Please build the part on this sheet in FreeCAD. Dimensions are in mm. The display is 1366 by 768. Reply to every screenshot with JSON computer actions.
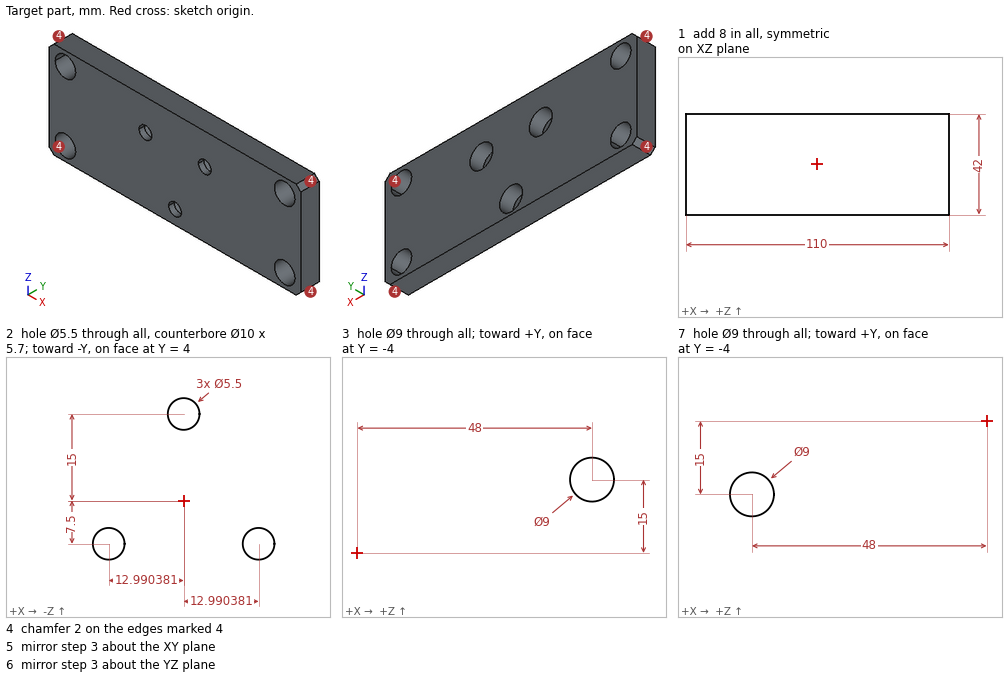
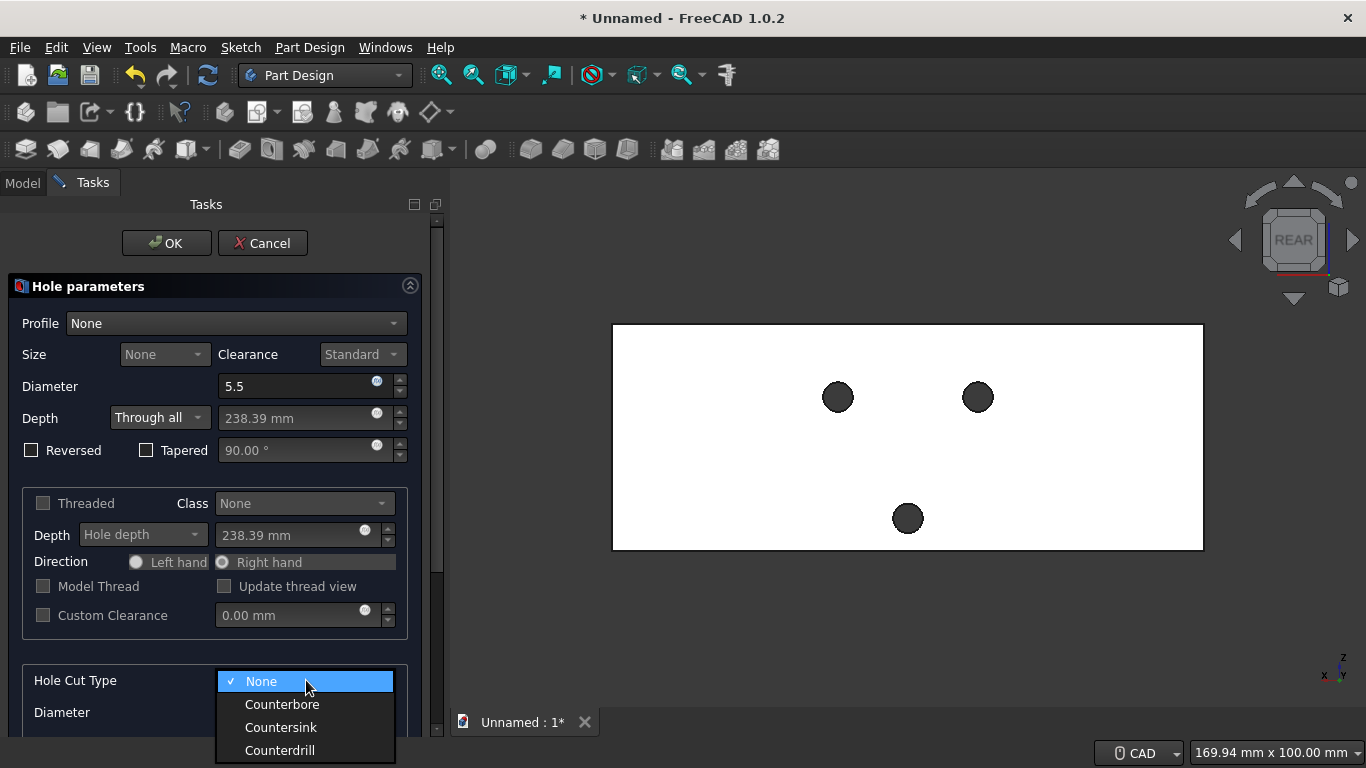
{"action": "left_click", "coordinate": [304, 704]}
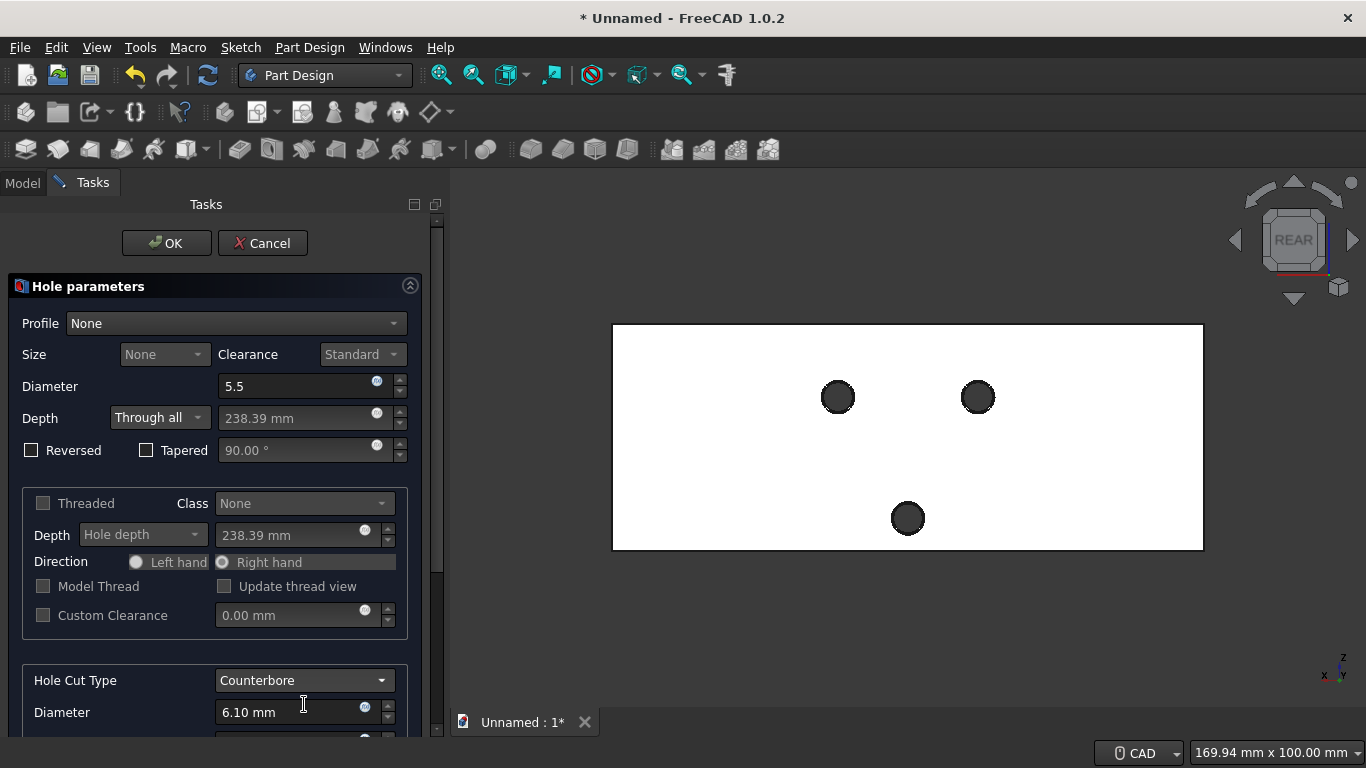
{"action": "triple_click", "coordinate": [298, 712]}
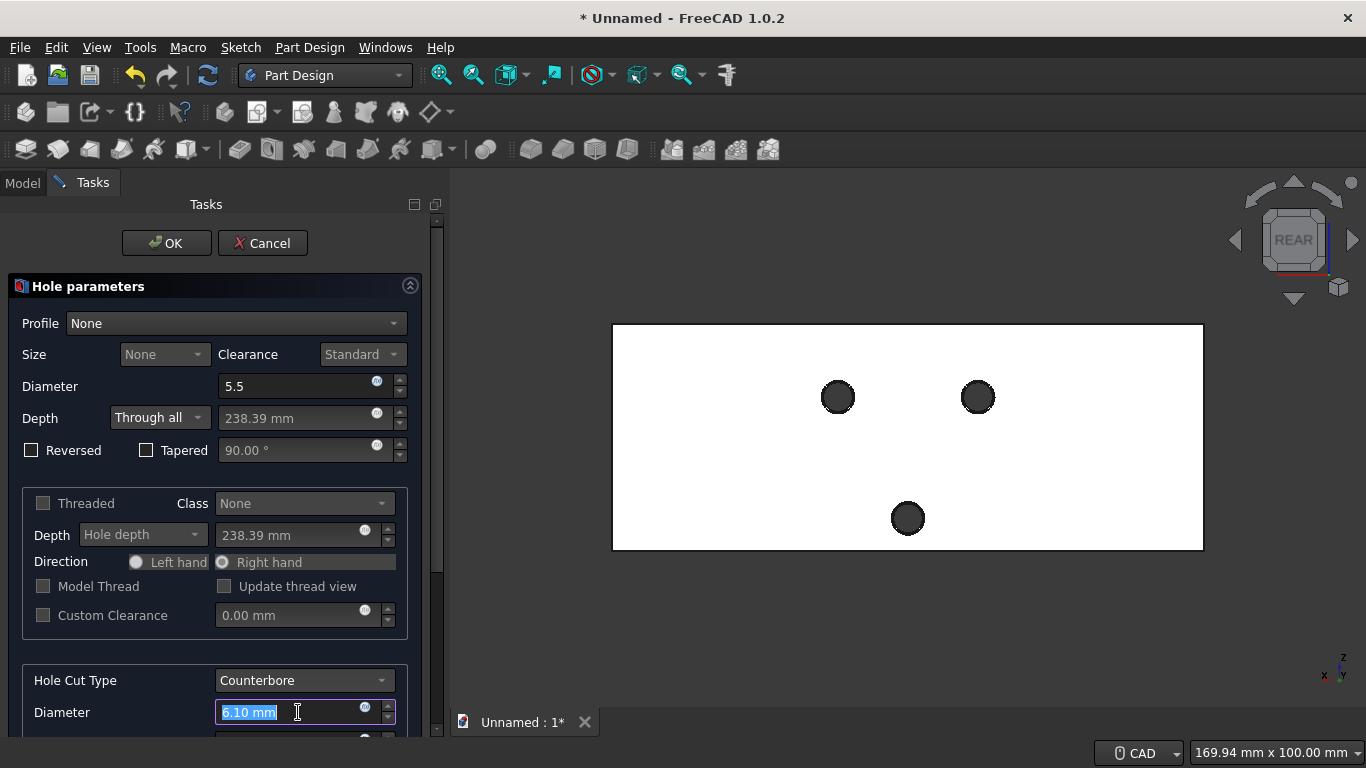
{"action": "type", "text": "10"}
{"action": "key", "text": "Tab"}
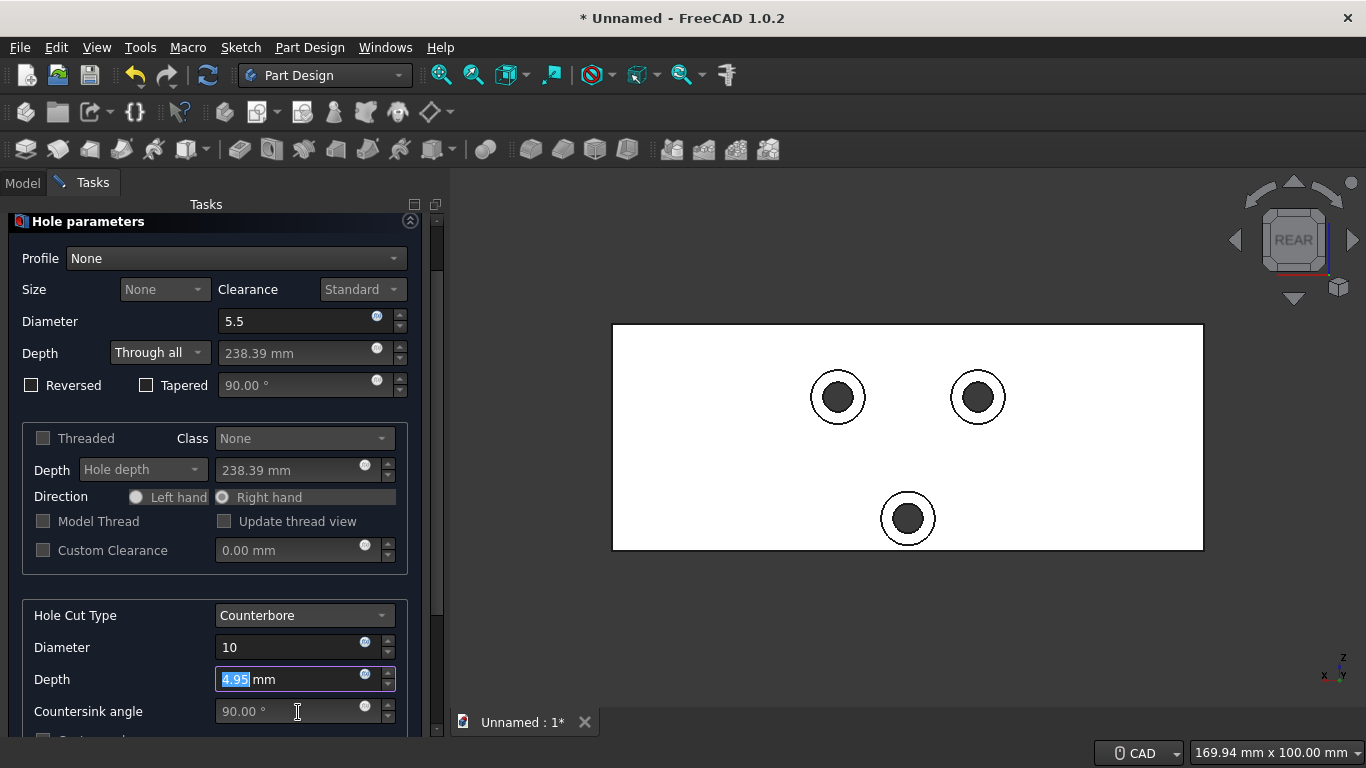
{"action": "type", "text": "5.7"}
{"action": "key", "text": "Tab"}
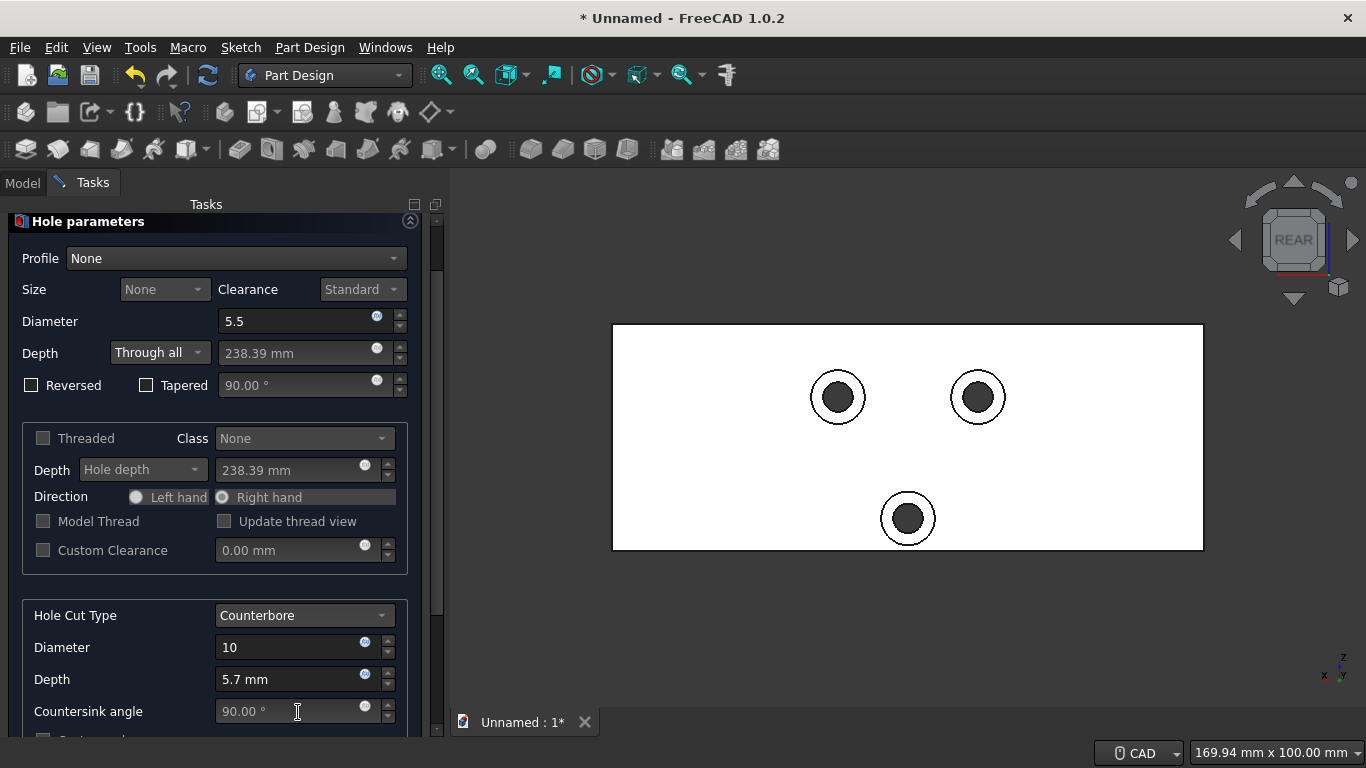
{"action": "scroll", "coordinate": [437, 475], "scroll_direction": "up", "scroll_amount": 2}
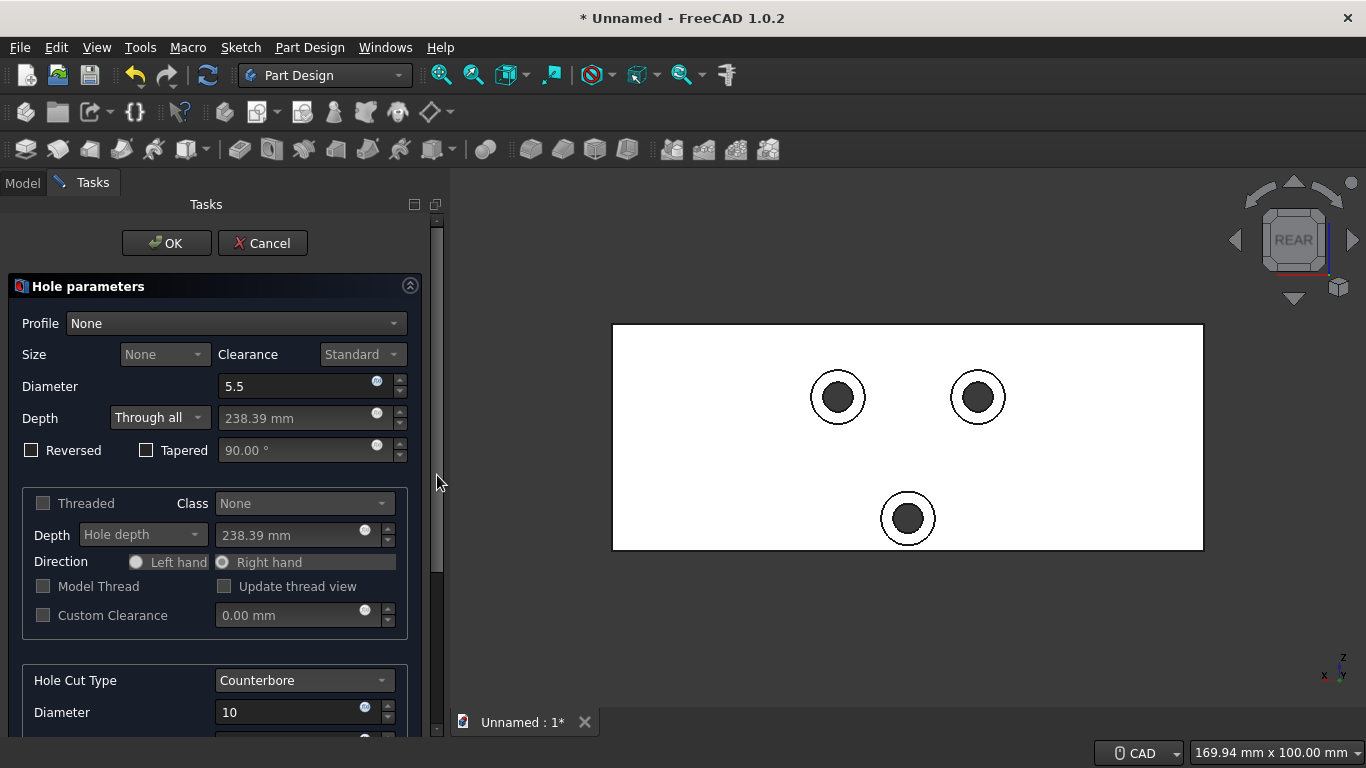
{"action": "left_click", "coordinate": [167, 243]}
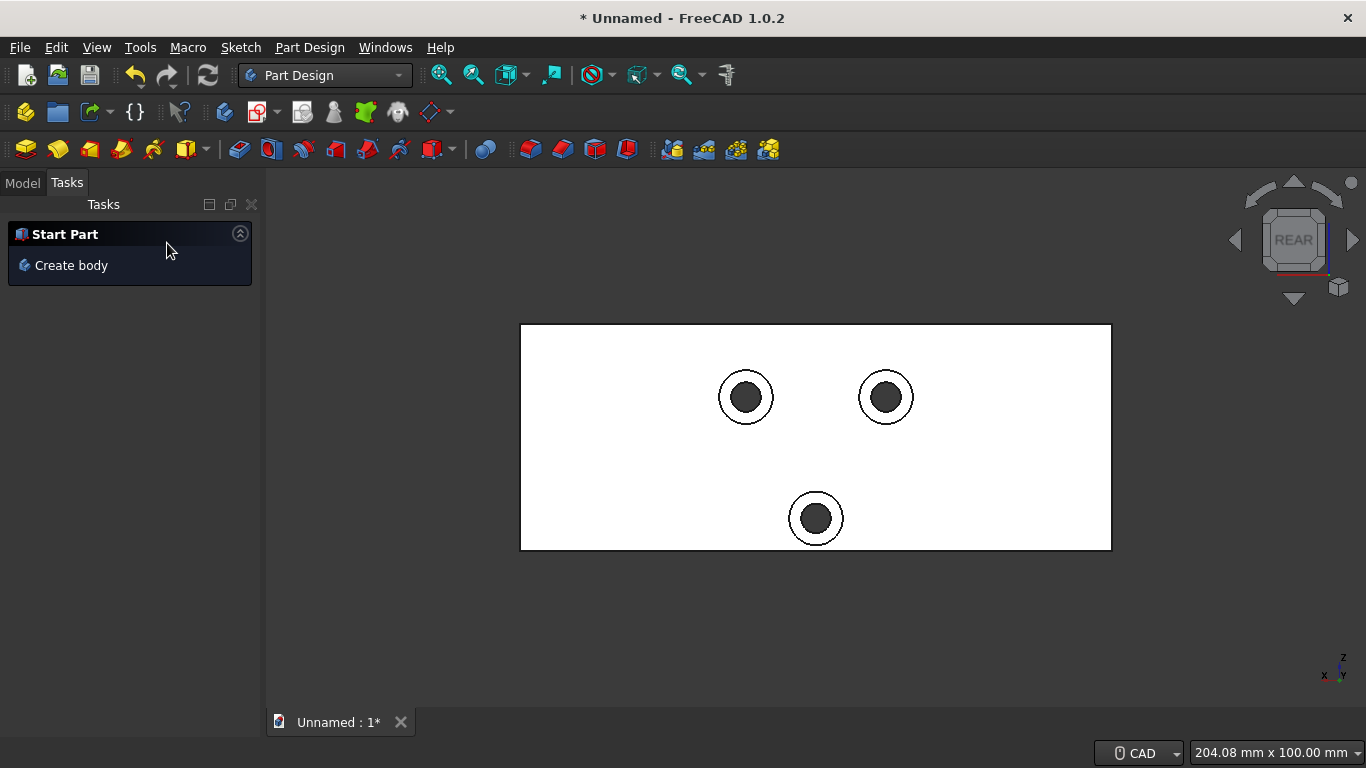
{"action": "key", "text": "0"}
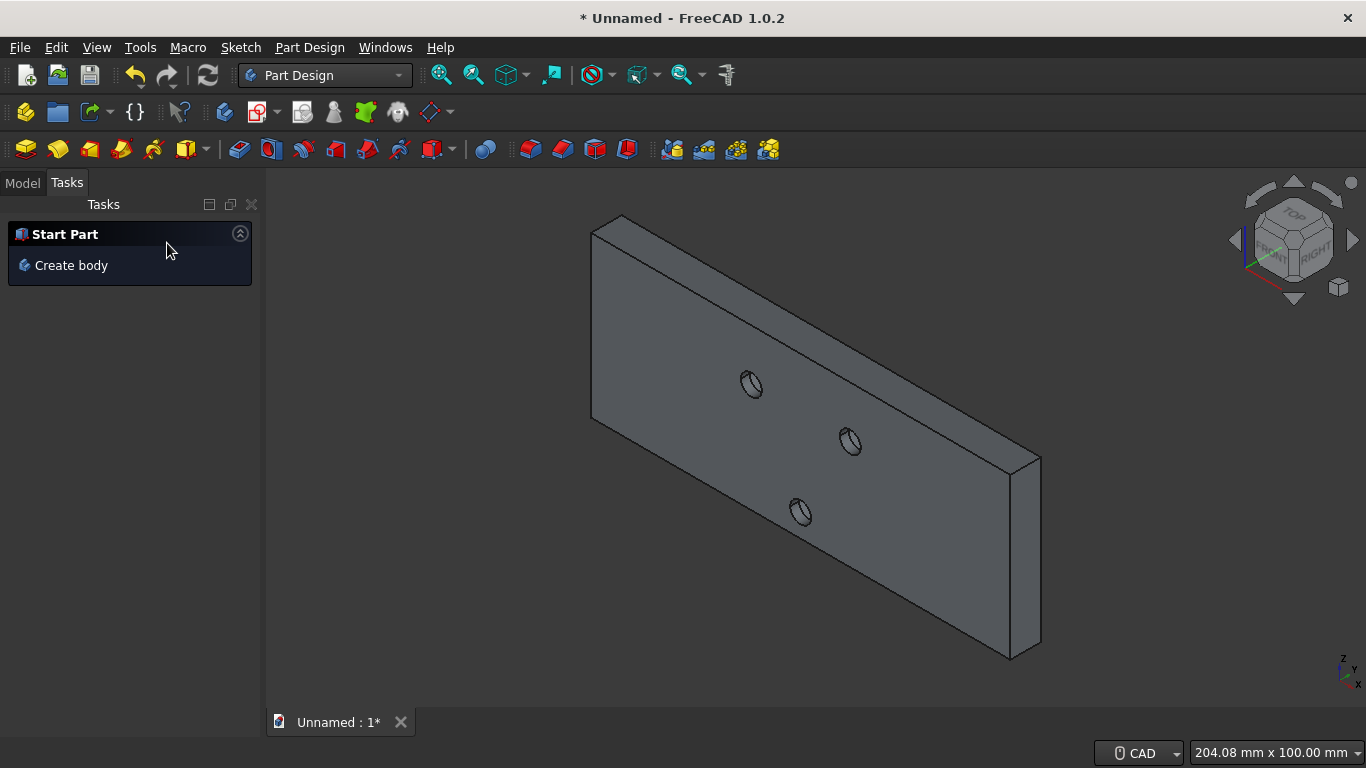
{"action": "left_click", "coordinate": [921, 514]}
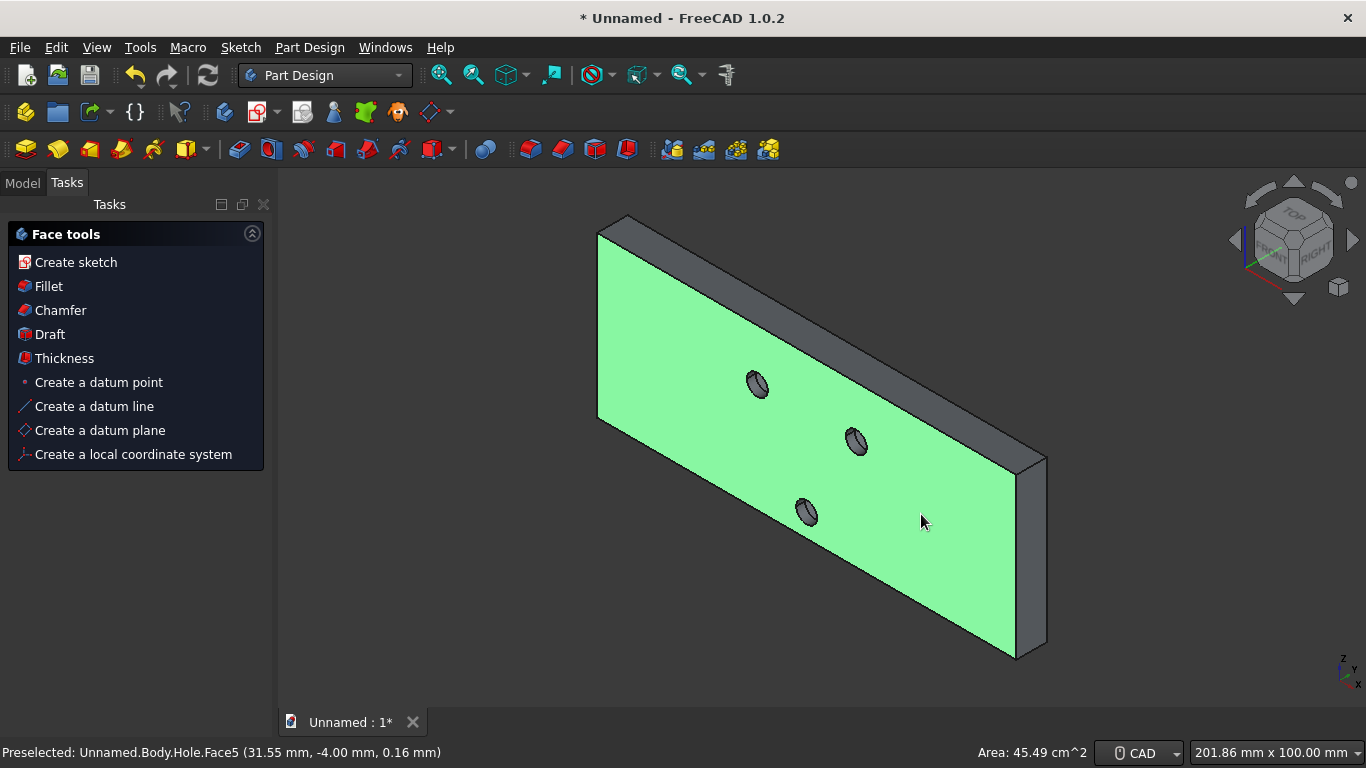
{"action": "left_click", "coordinate": [258, 112]}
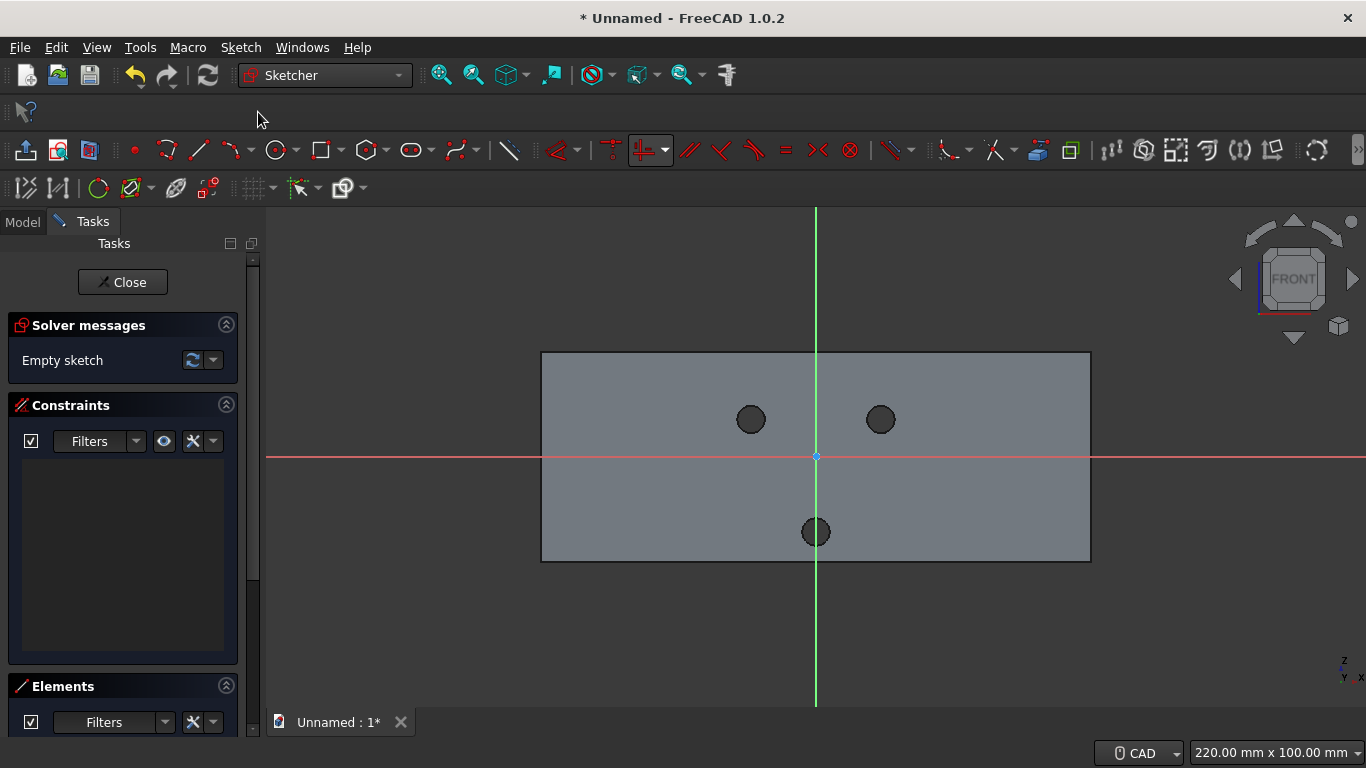
{"action": "scroll", "coordinate": [1104, 370], "scroll_direction": "up", "scroll_amount": 10}